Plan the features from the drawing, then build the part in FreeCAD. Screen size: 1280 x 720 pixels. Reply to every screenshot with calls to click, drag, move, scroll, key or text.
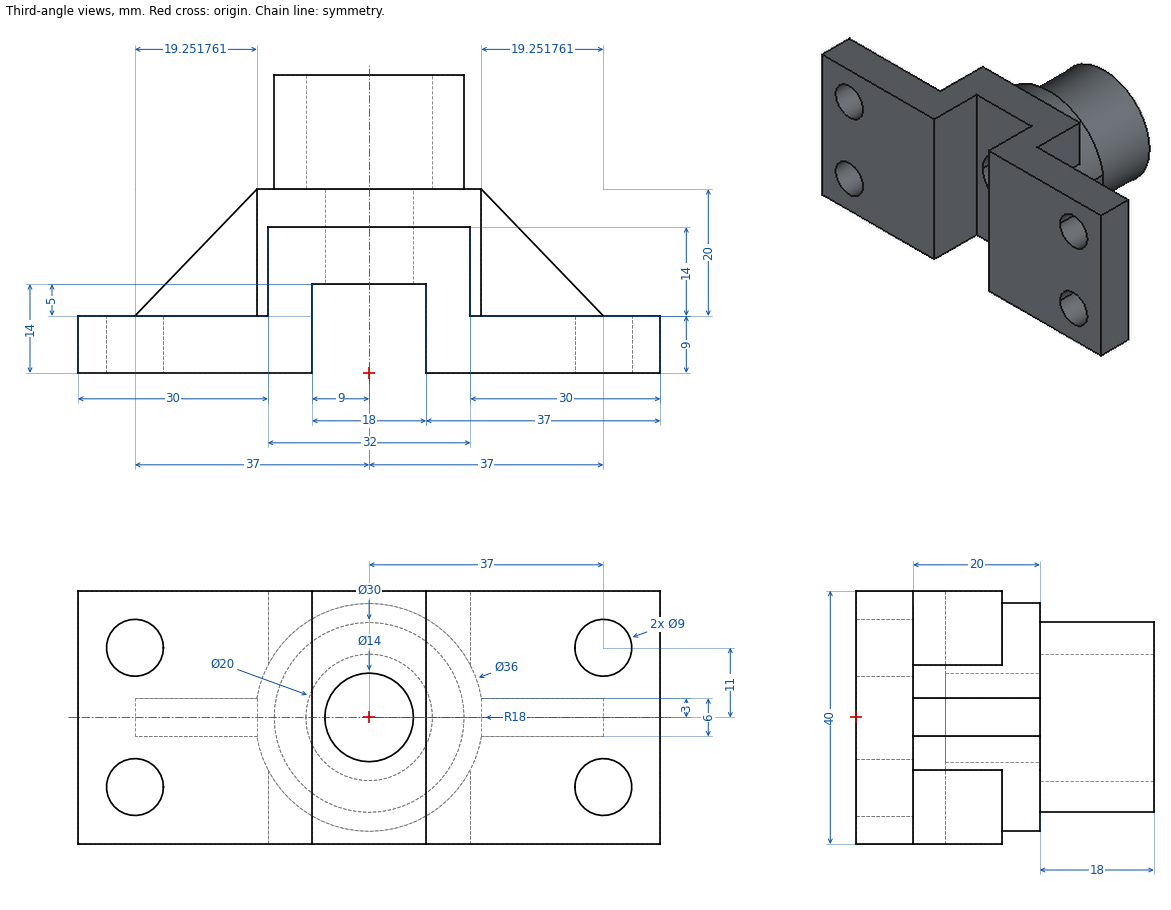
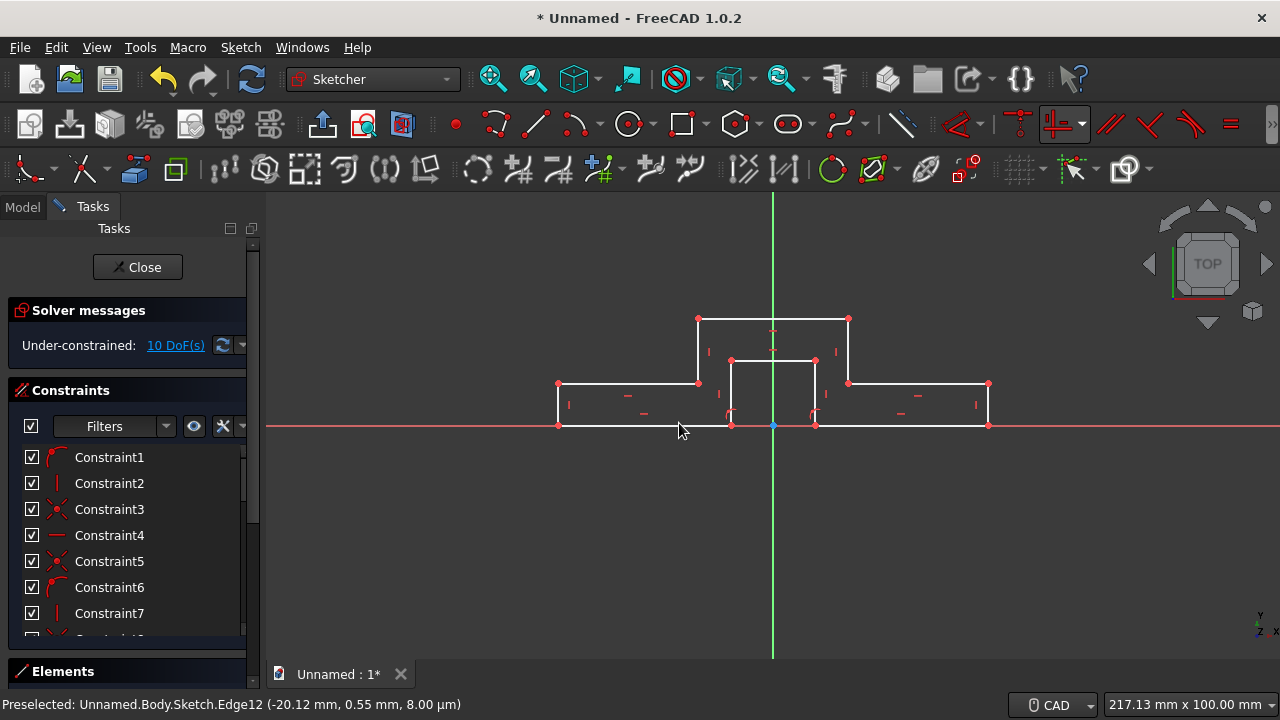
click(848, 384)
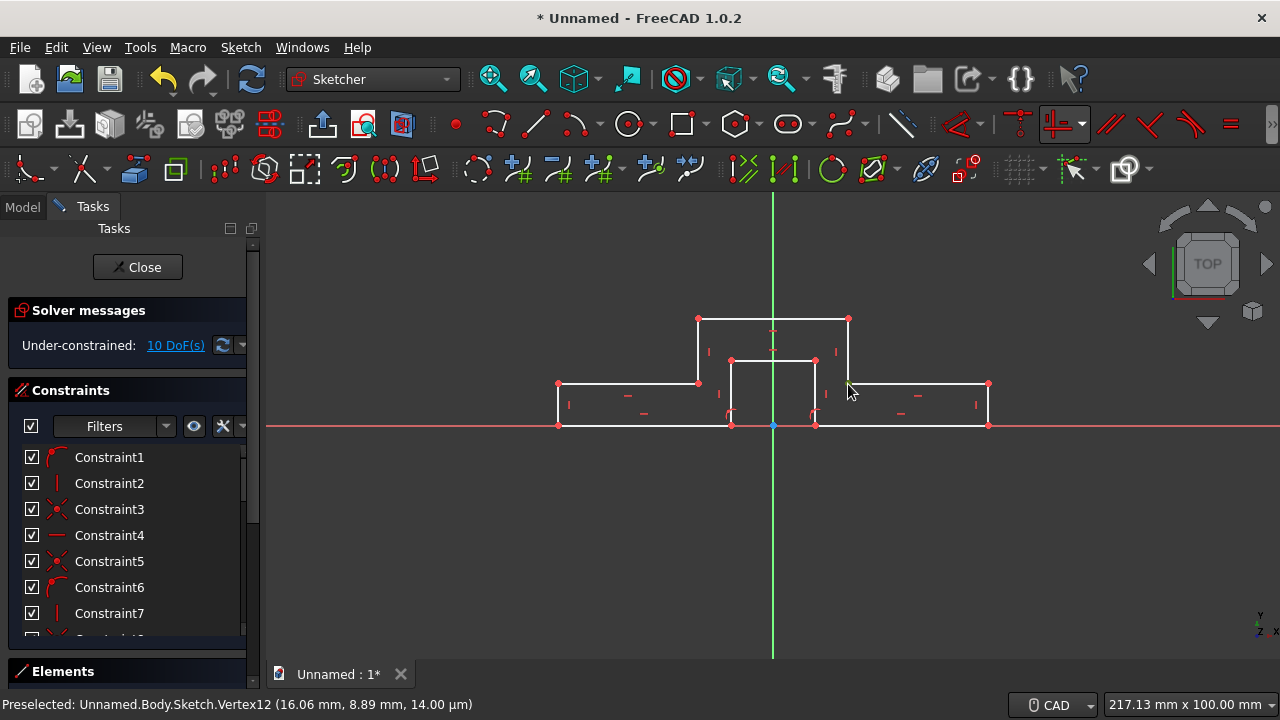
click(698, 384)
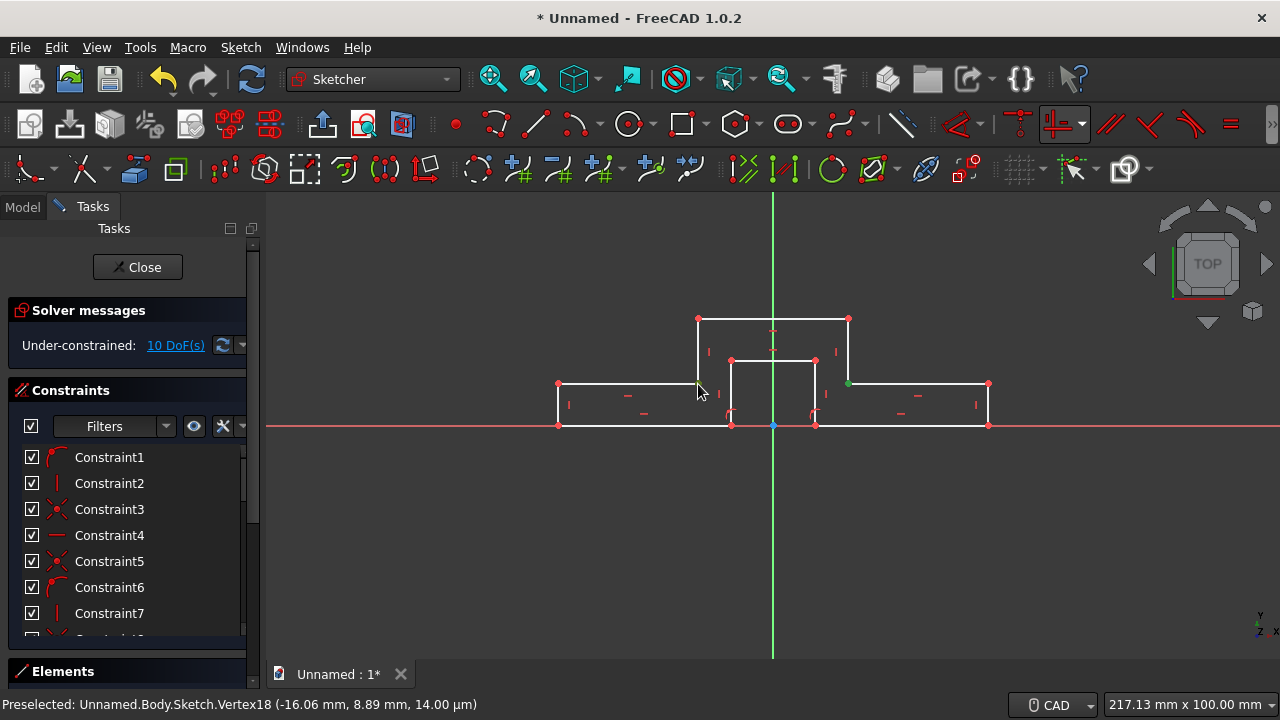
click(773, 602)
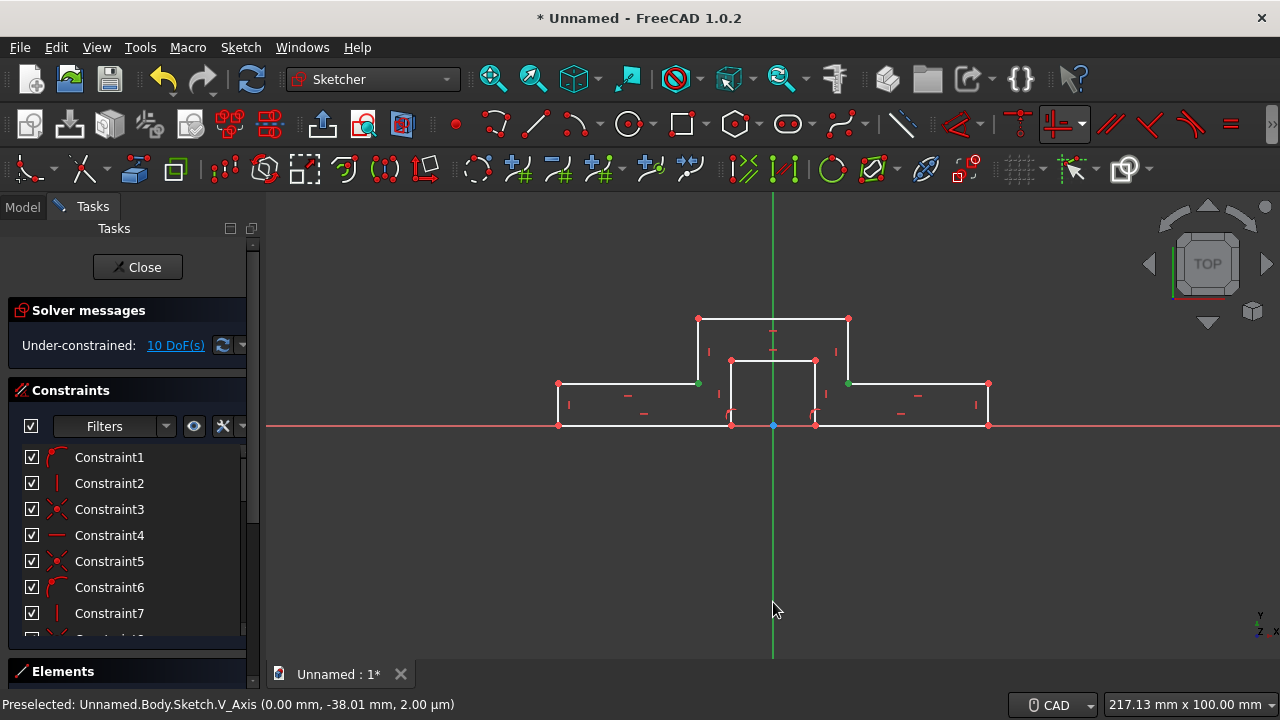
key(s)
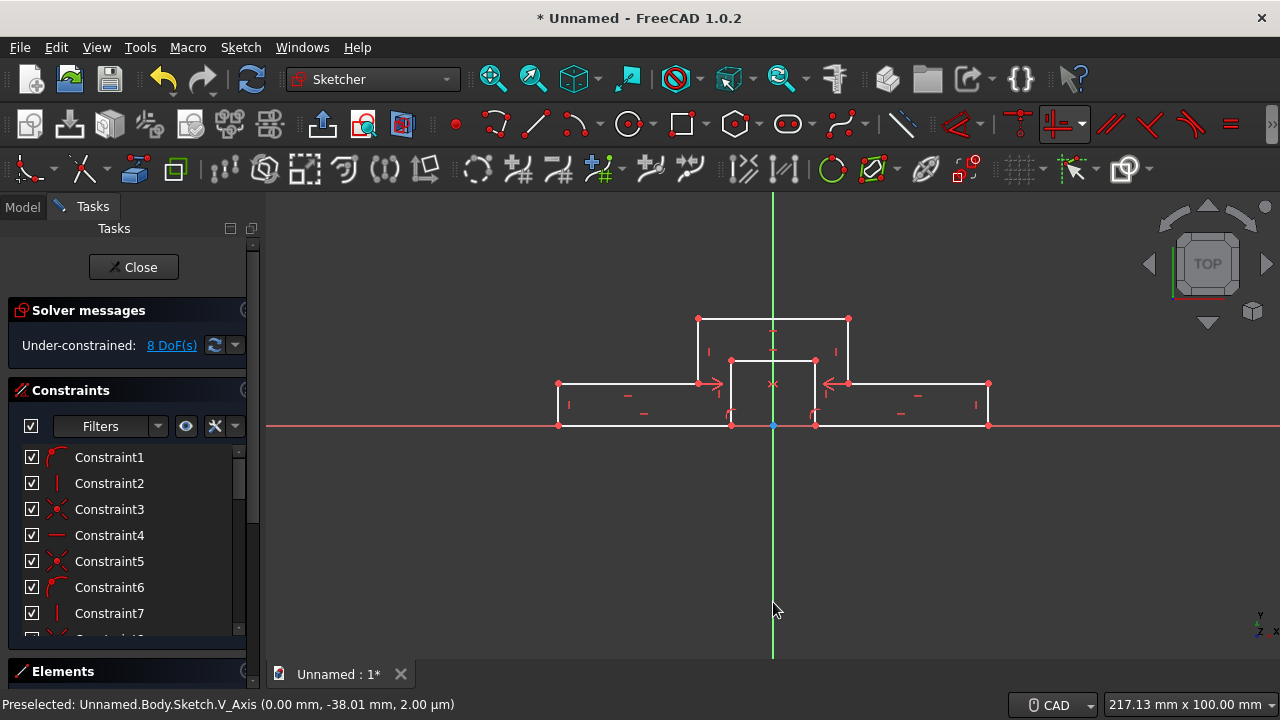
key(d)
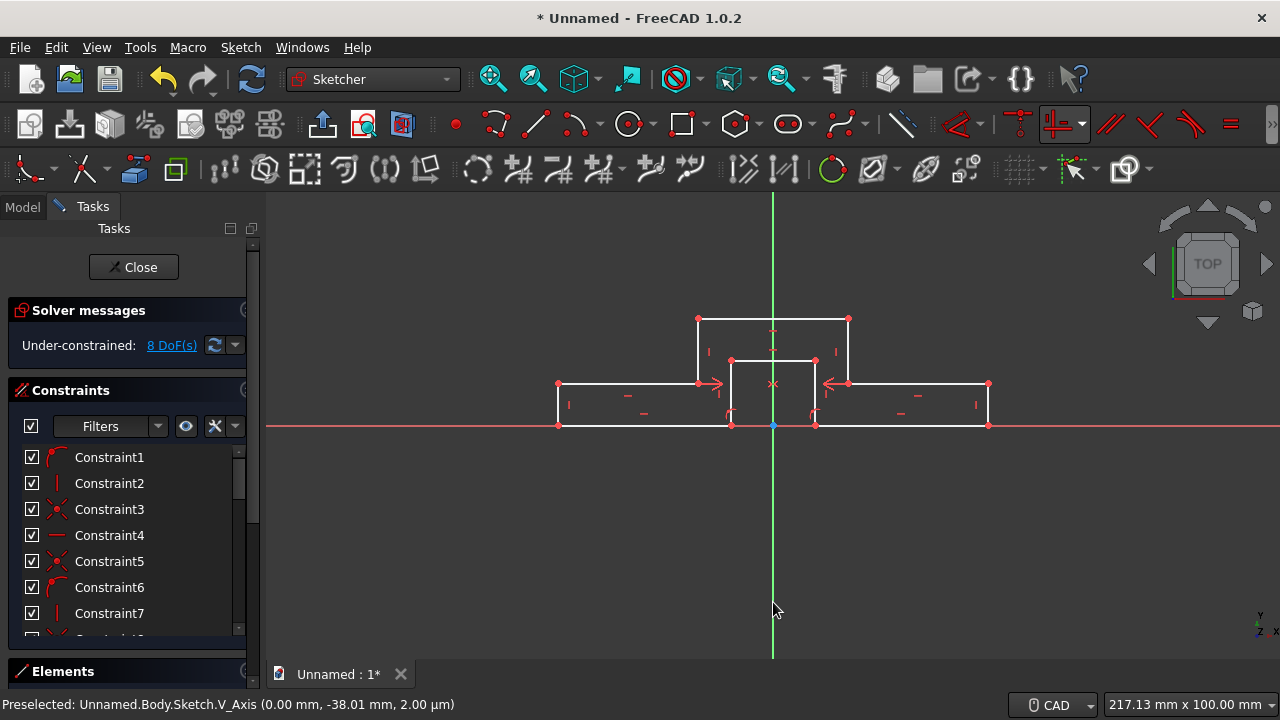
click(988, 413)
click(1022, 405)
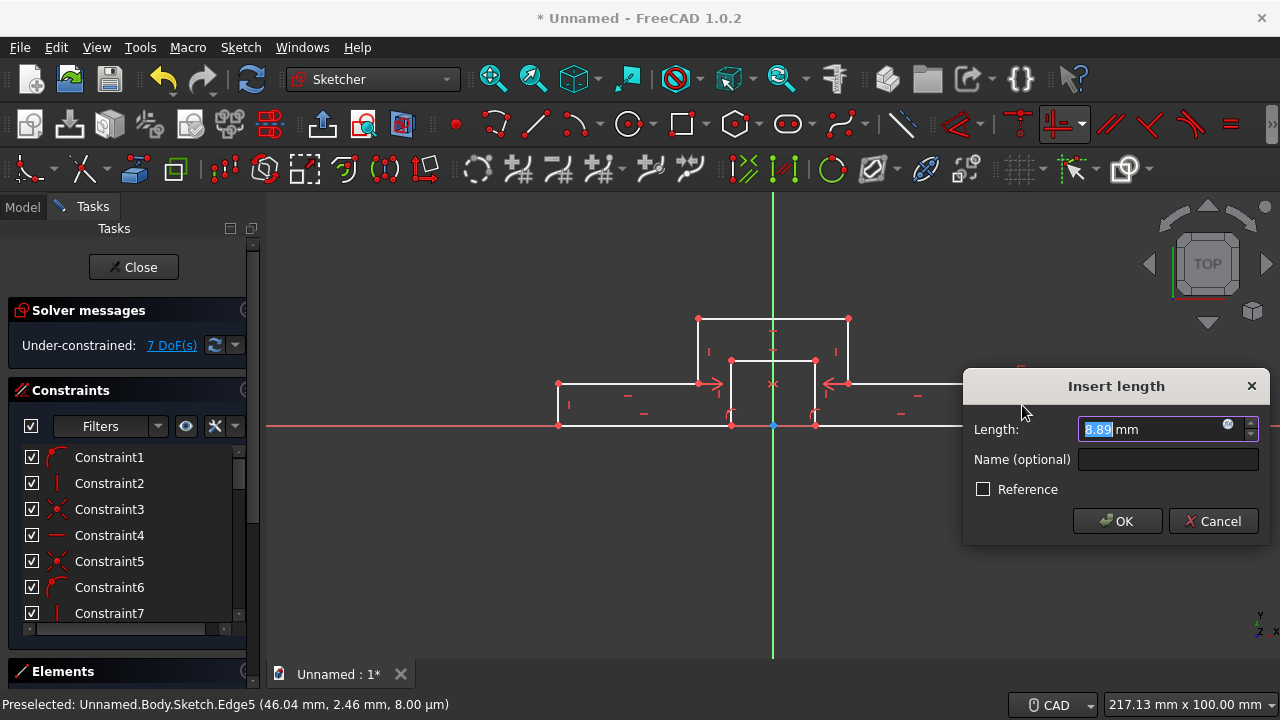
text(9)
key(Return)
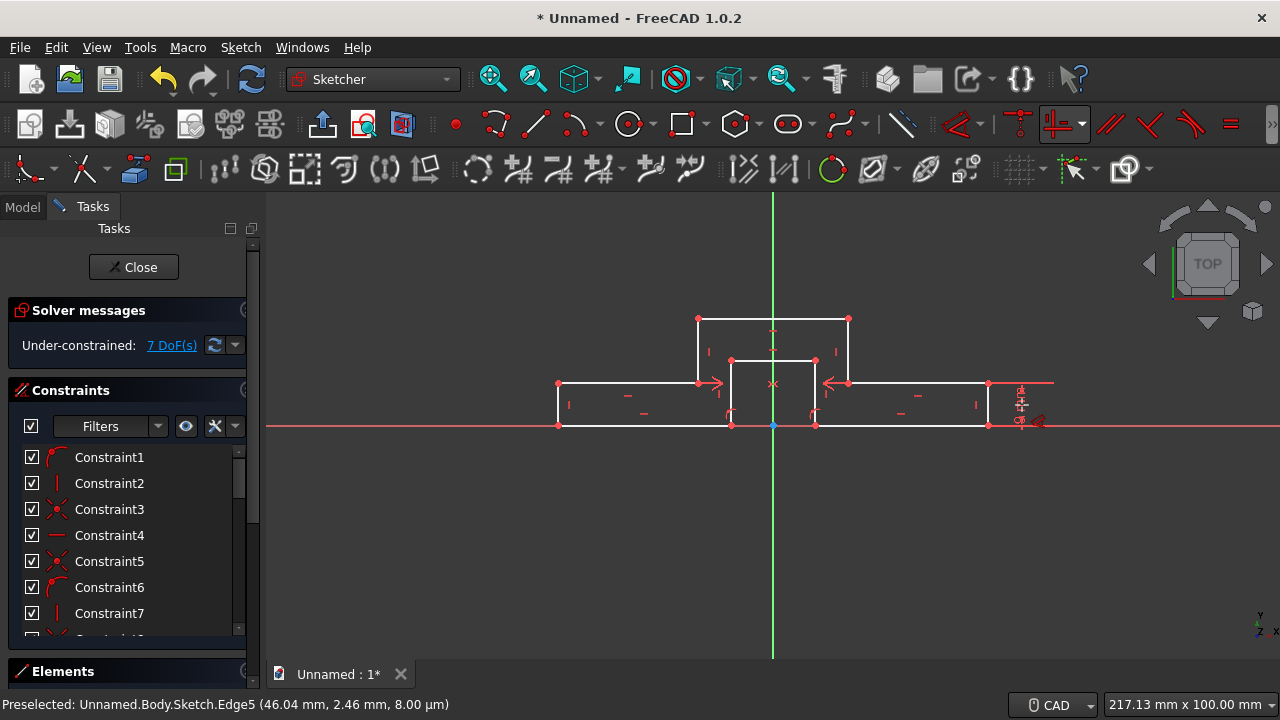
click(731, 406)
click(697, 408)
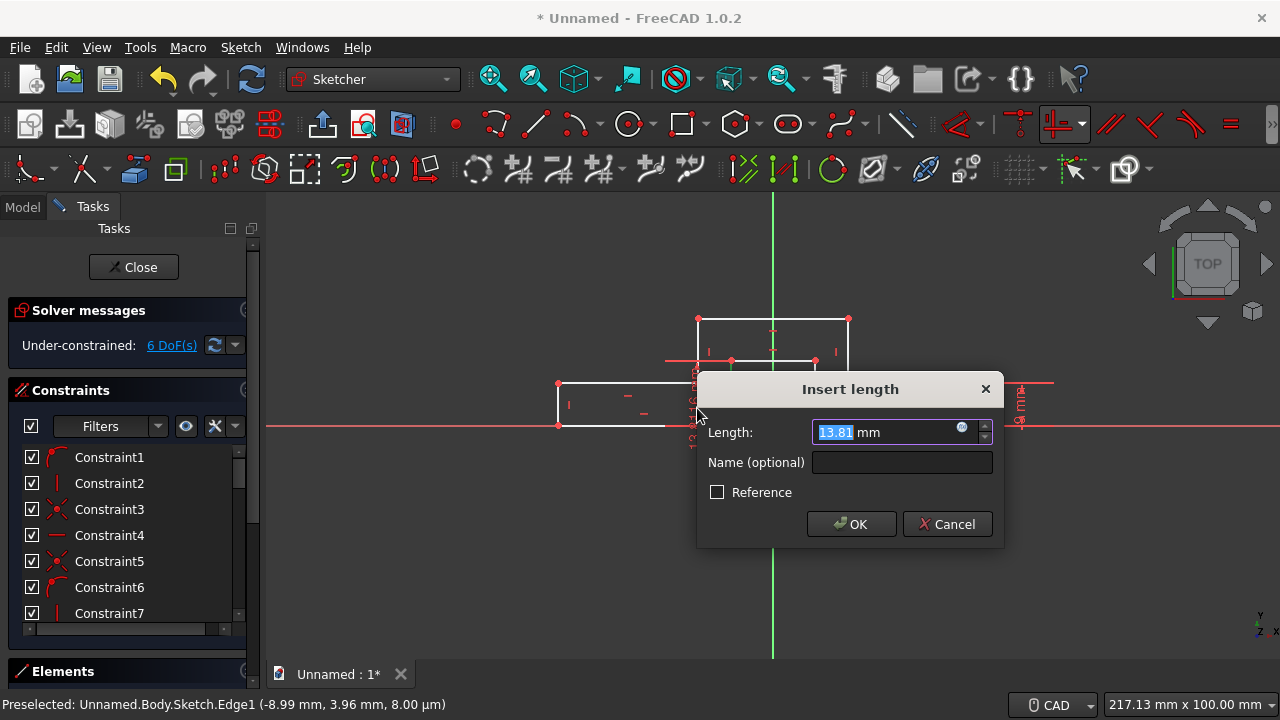
text(14)
key(Return)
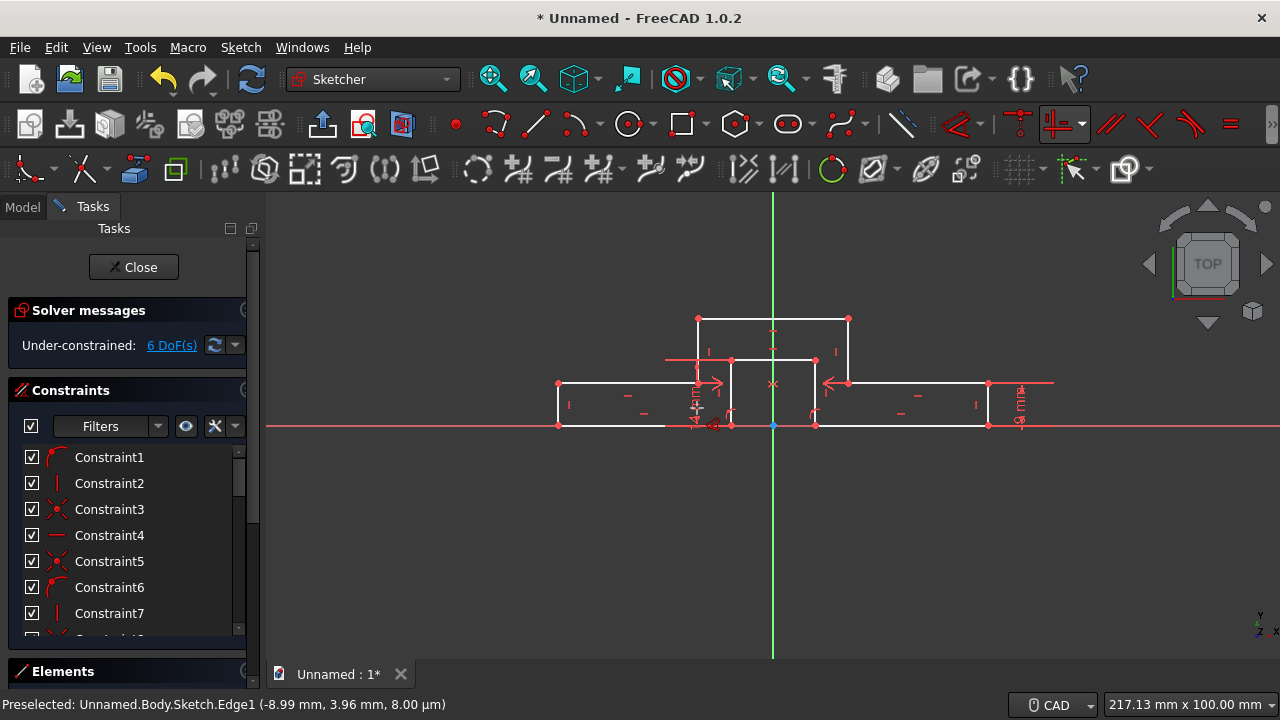
click(756, 360)
click(792, 394)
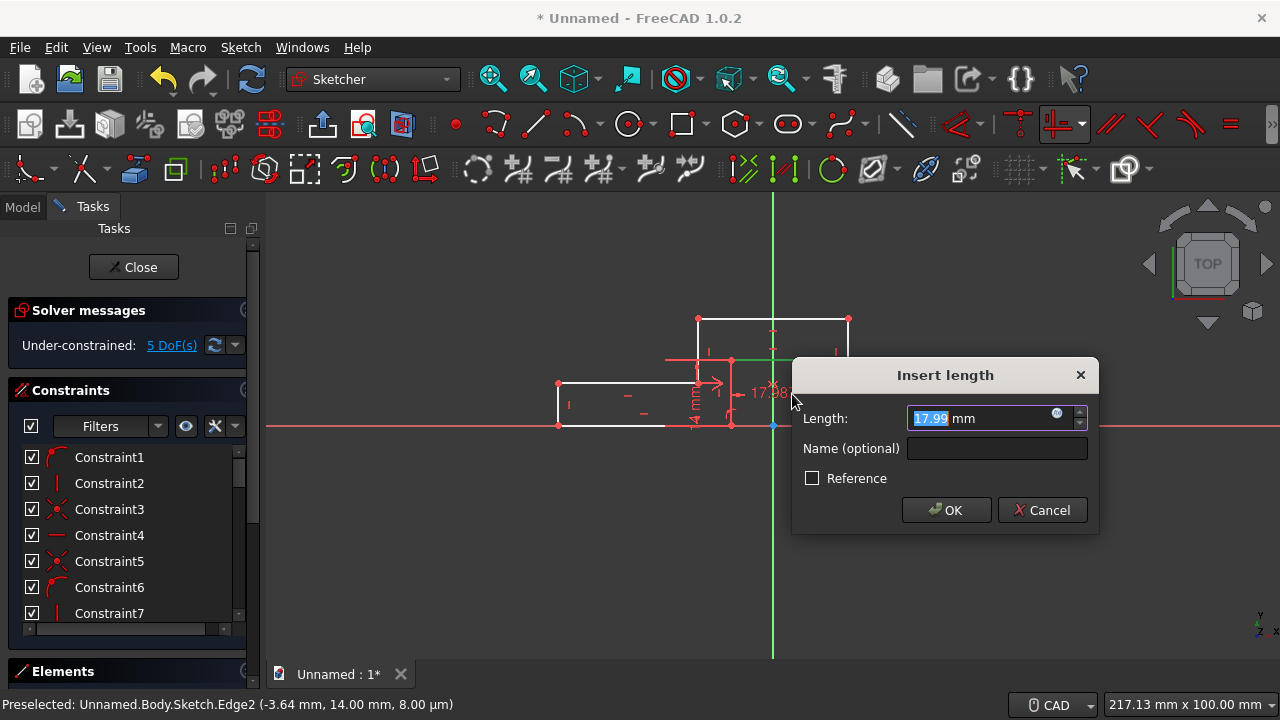
text(18)
key(Return)